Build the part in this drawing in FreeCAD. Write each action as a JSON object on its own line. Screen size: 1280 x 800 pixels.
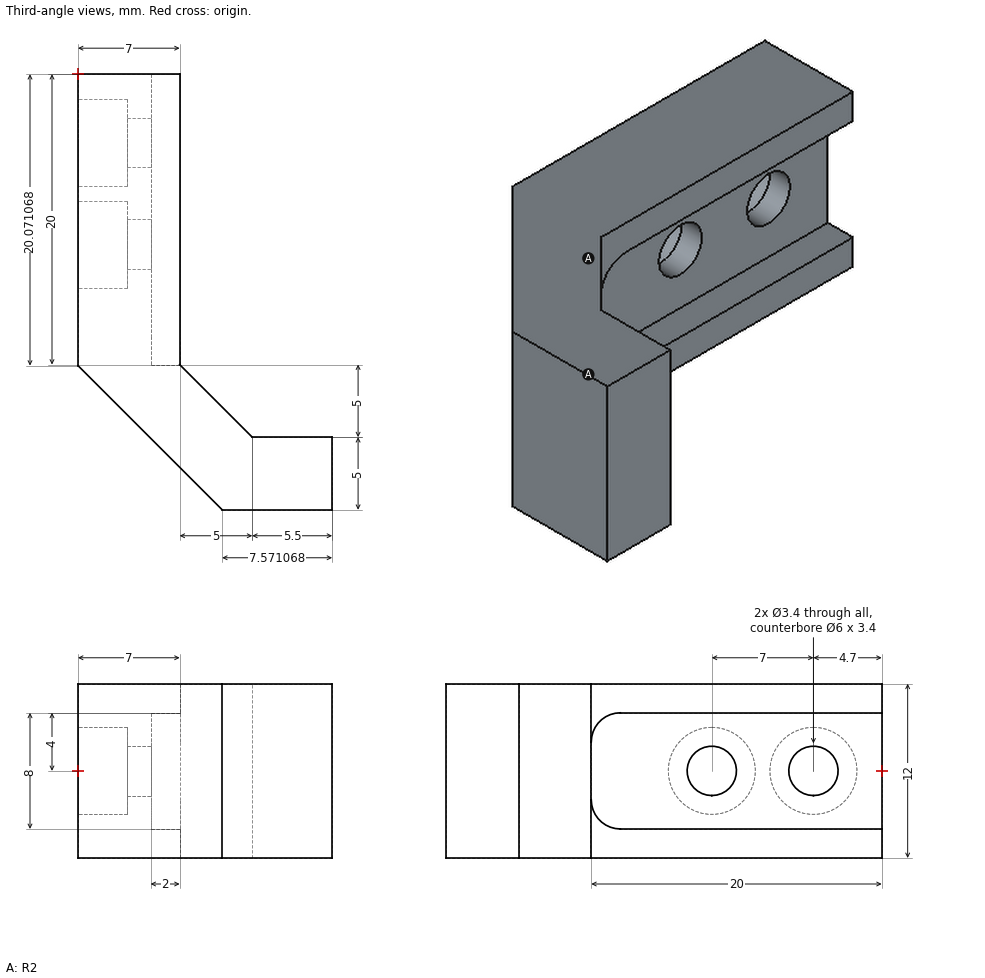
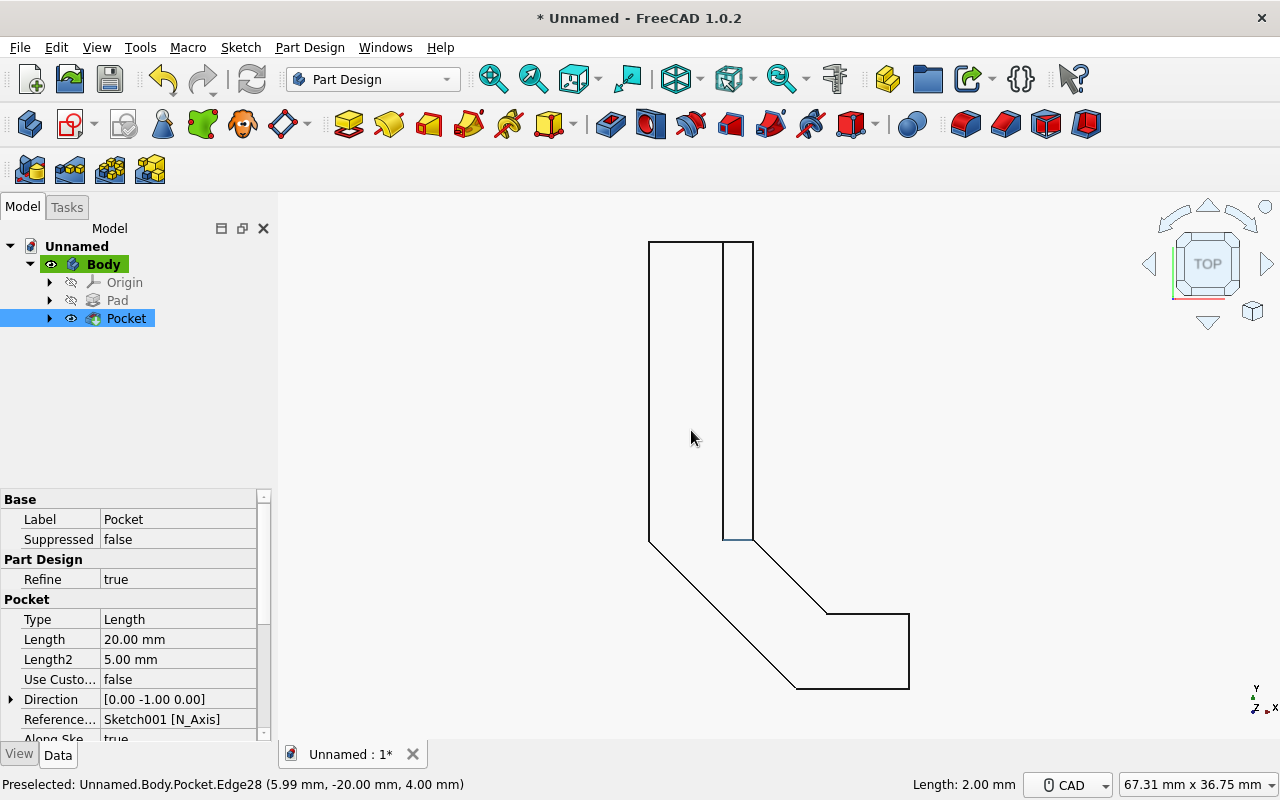
{"action": "key", "text": "1"}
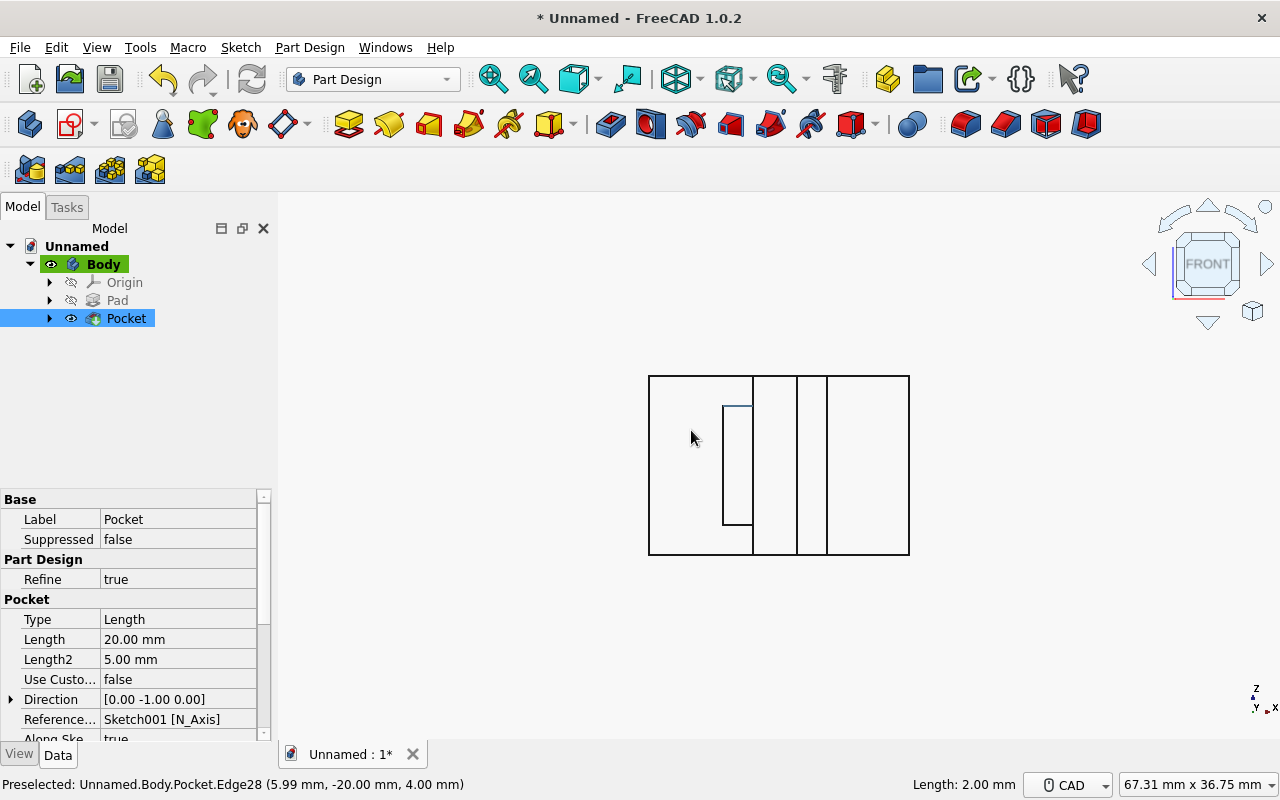
{"action": "left_click", "coordinate": [494, 80]}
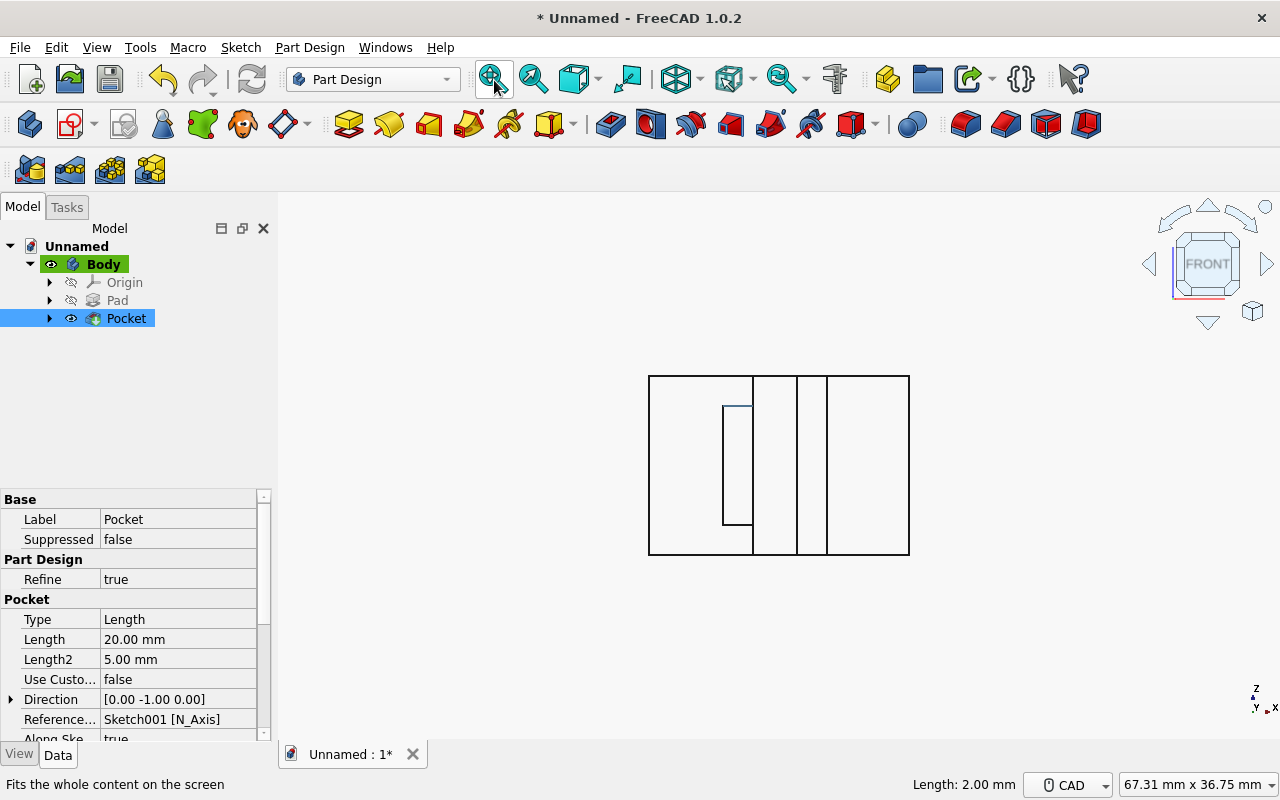
{"action": "left_click", "coordinate": [738, 524], "text": "ctrl"}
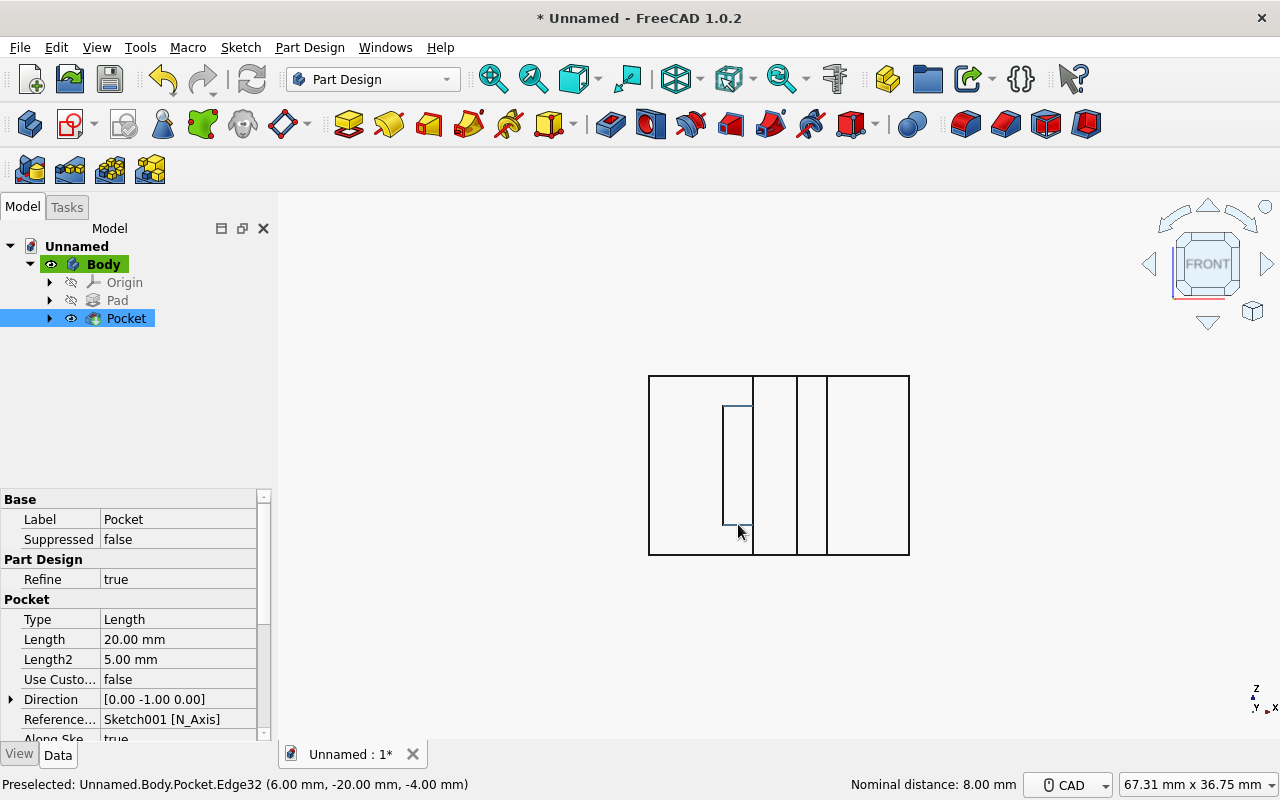
{"action": "key", "text": "v 1"}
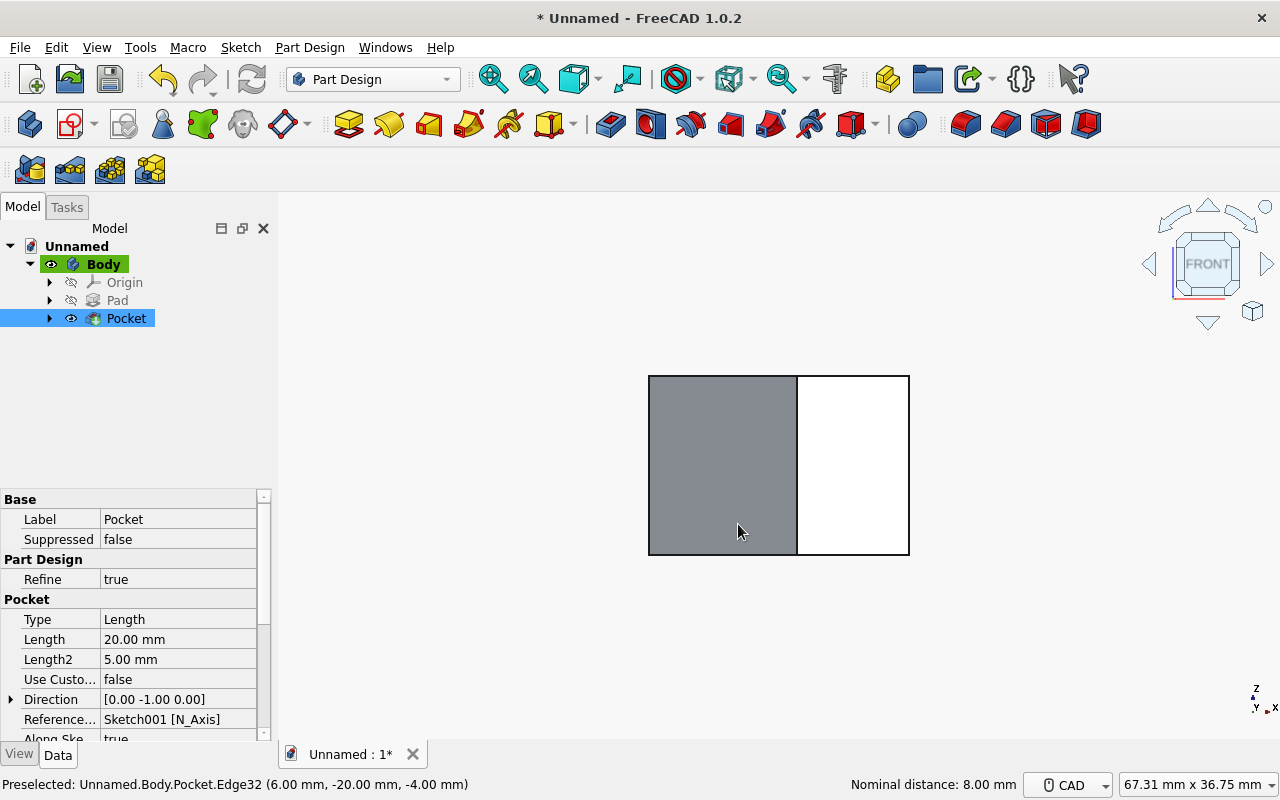
{"action": "left_click", "coordinate": [966, 124]}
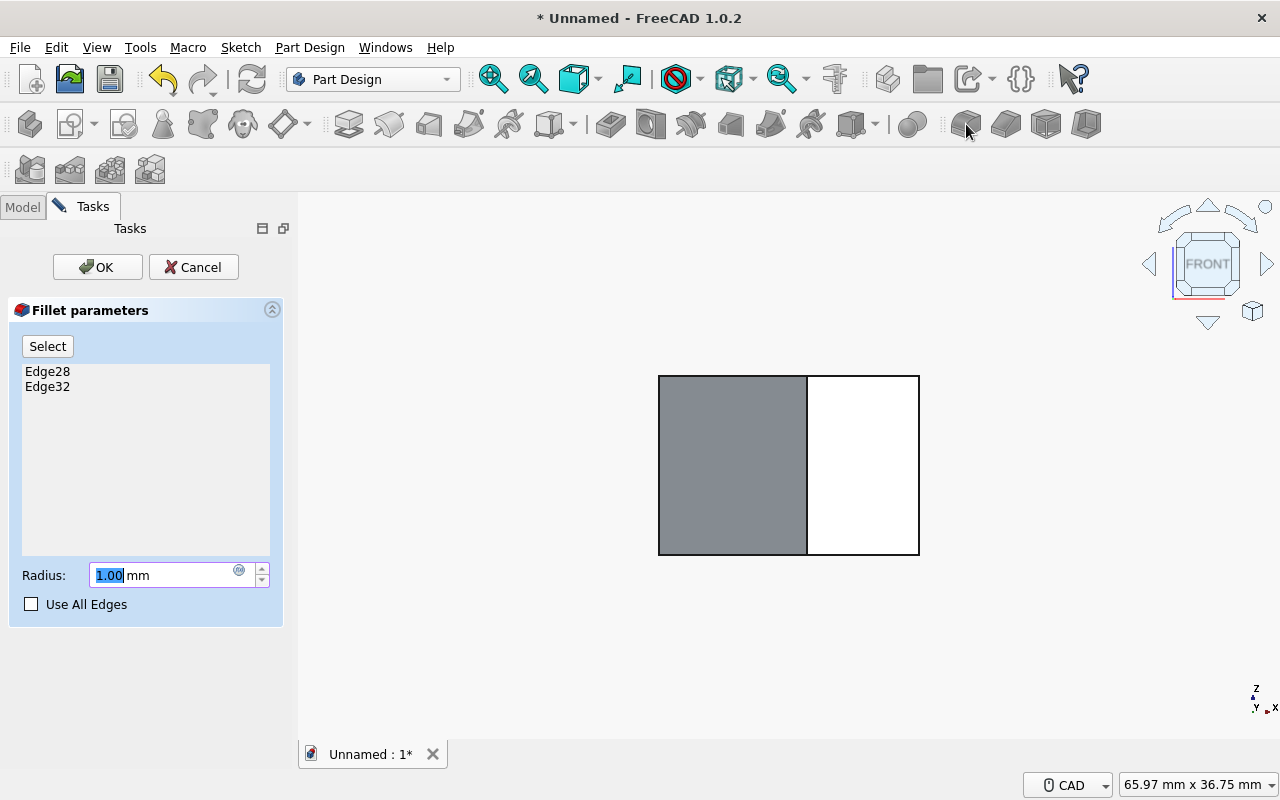
{"action": "type", "text": "2"}
{"action": "key", "text": "Tab"}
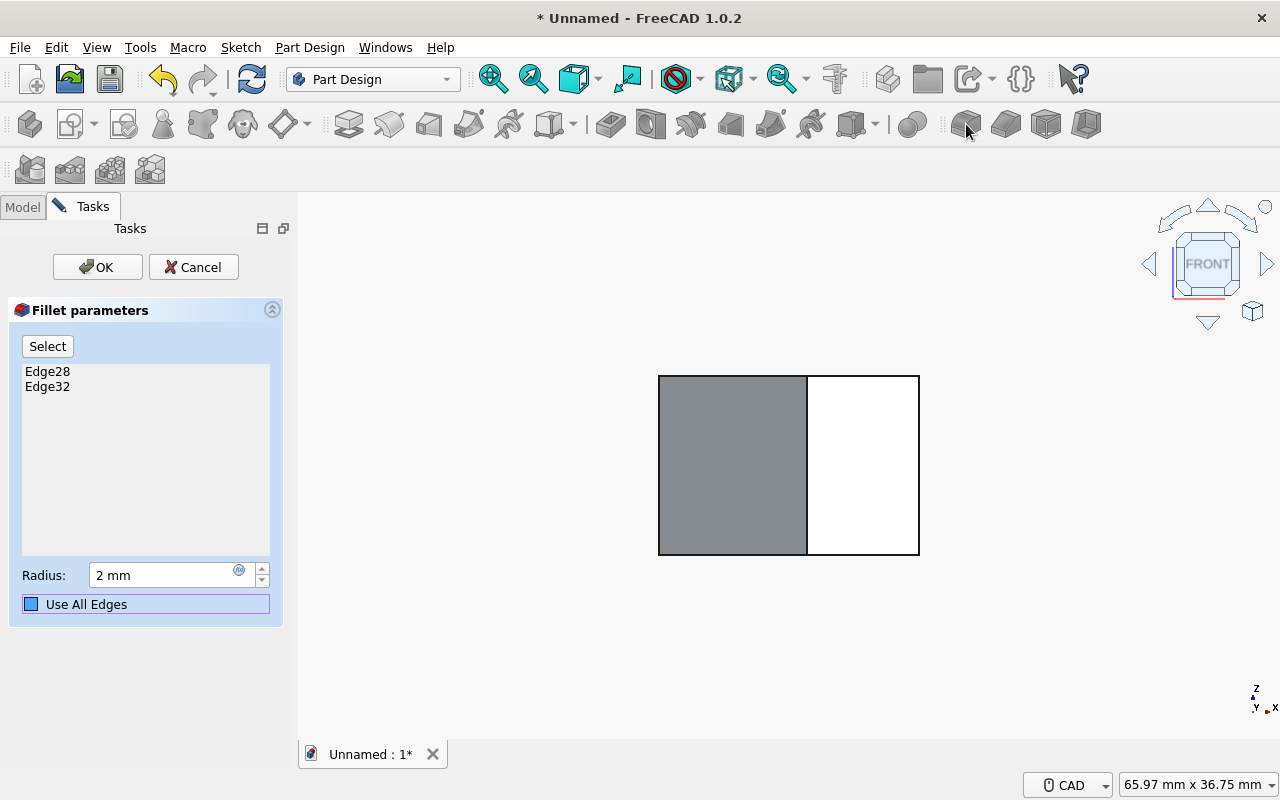
{"action": "left_click", "coordinate": [98, 267]}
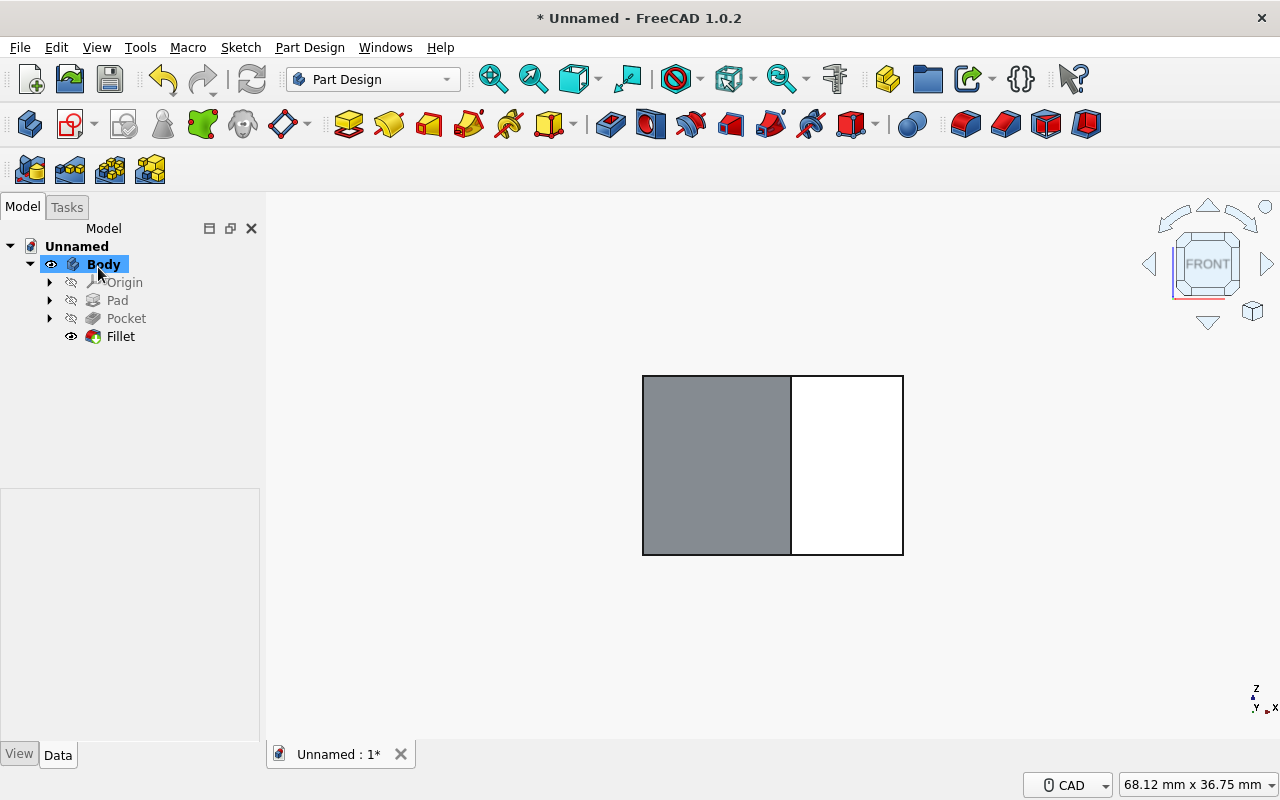
{"action": "left_click", "coordinate": [494, 80]}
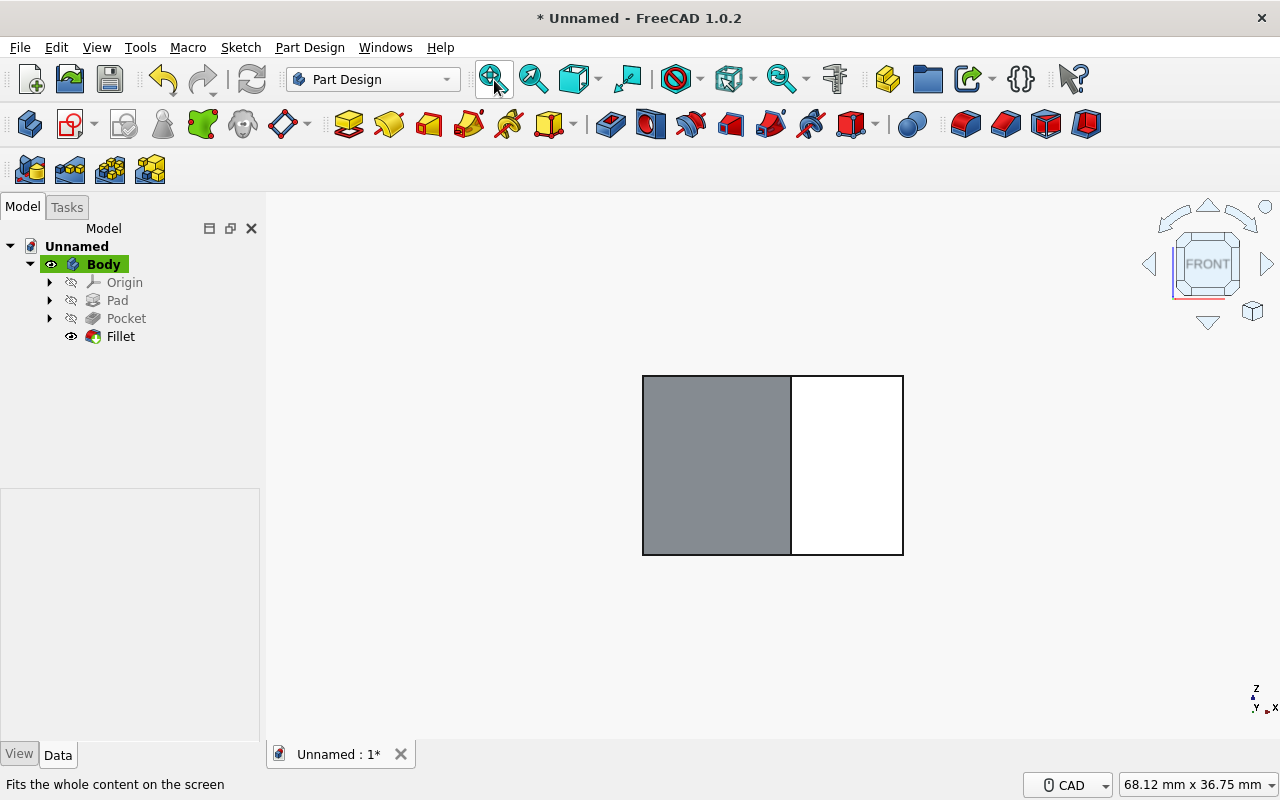
{"action": "key", "text": "6"}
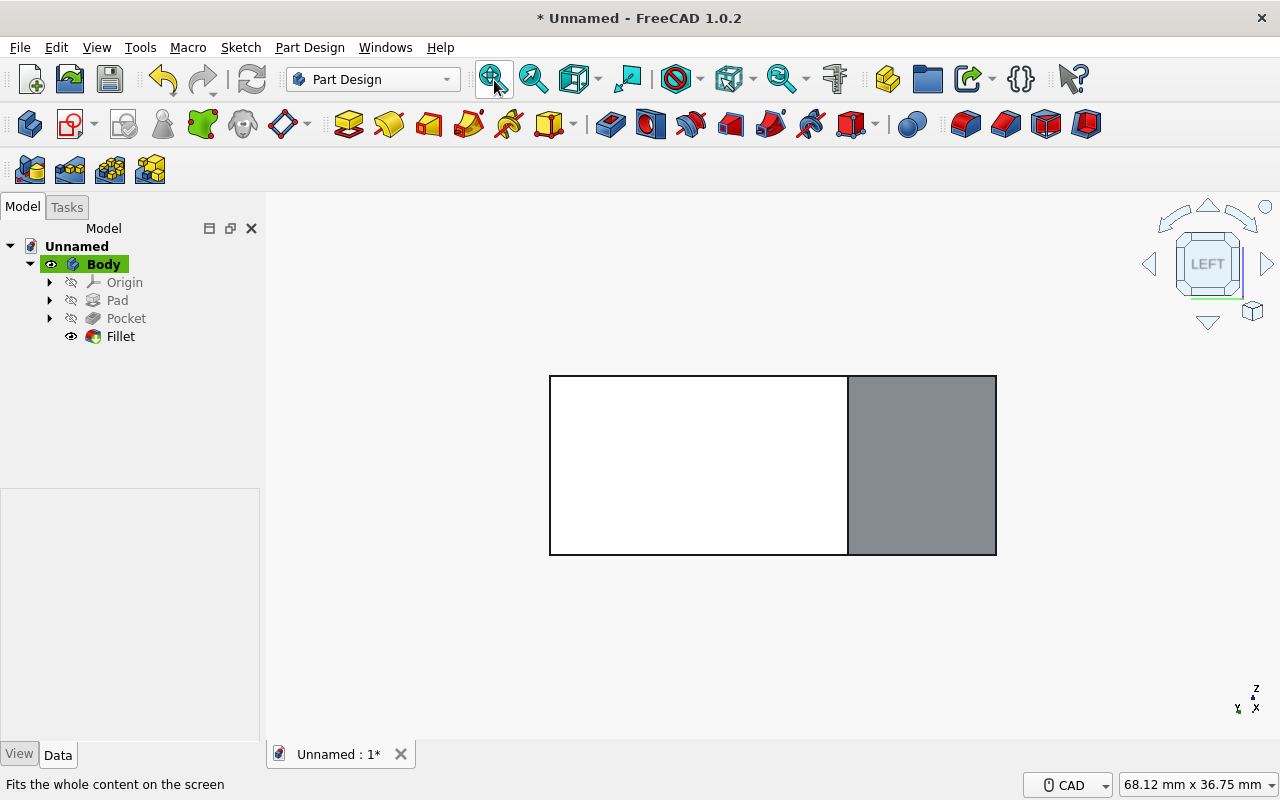
{"action": "left_click", "coordinate": [494, 80]}